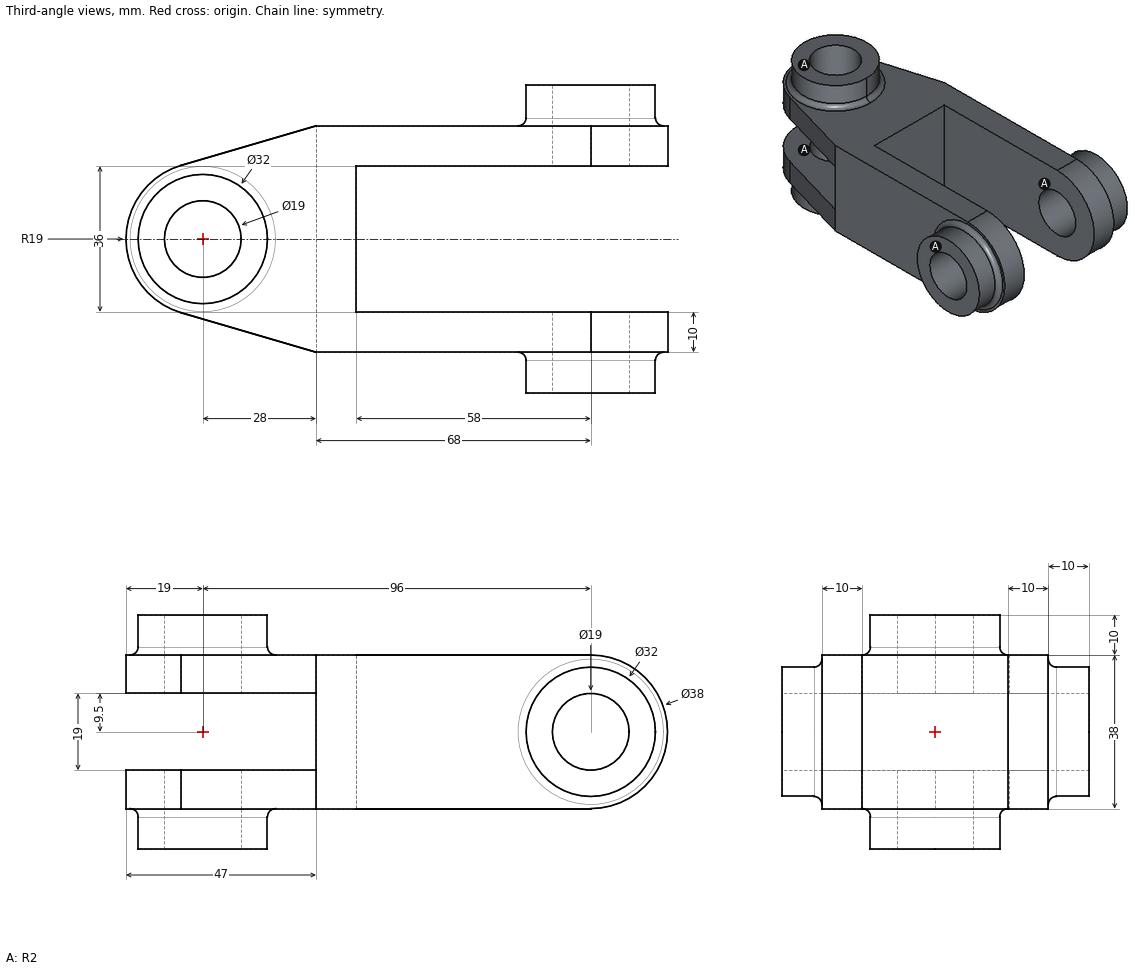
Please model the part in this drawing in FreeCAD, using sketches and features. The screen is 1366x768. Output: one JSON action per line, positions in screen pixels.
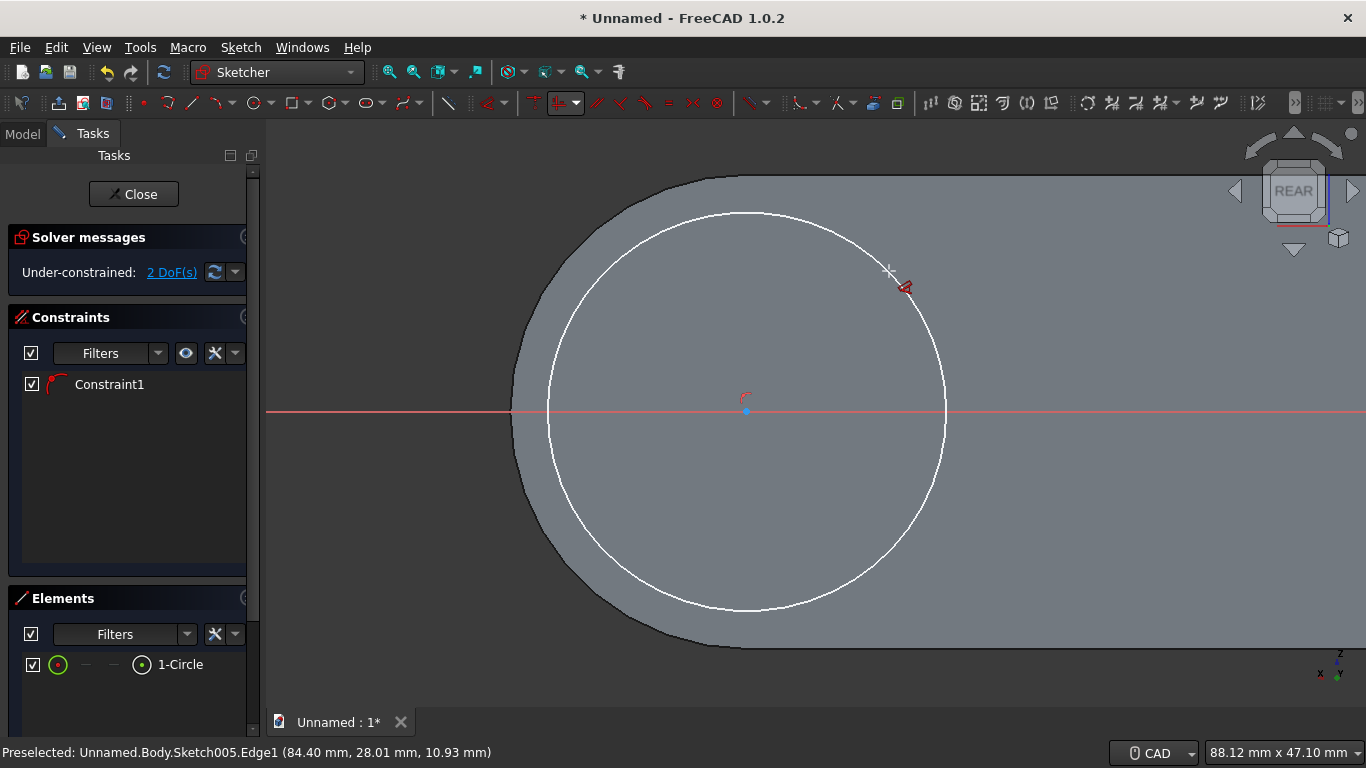
{"action": "left_click", "coordinate": [887, 270]}
{"action": "left_click", "coordinate": [909, 247]}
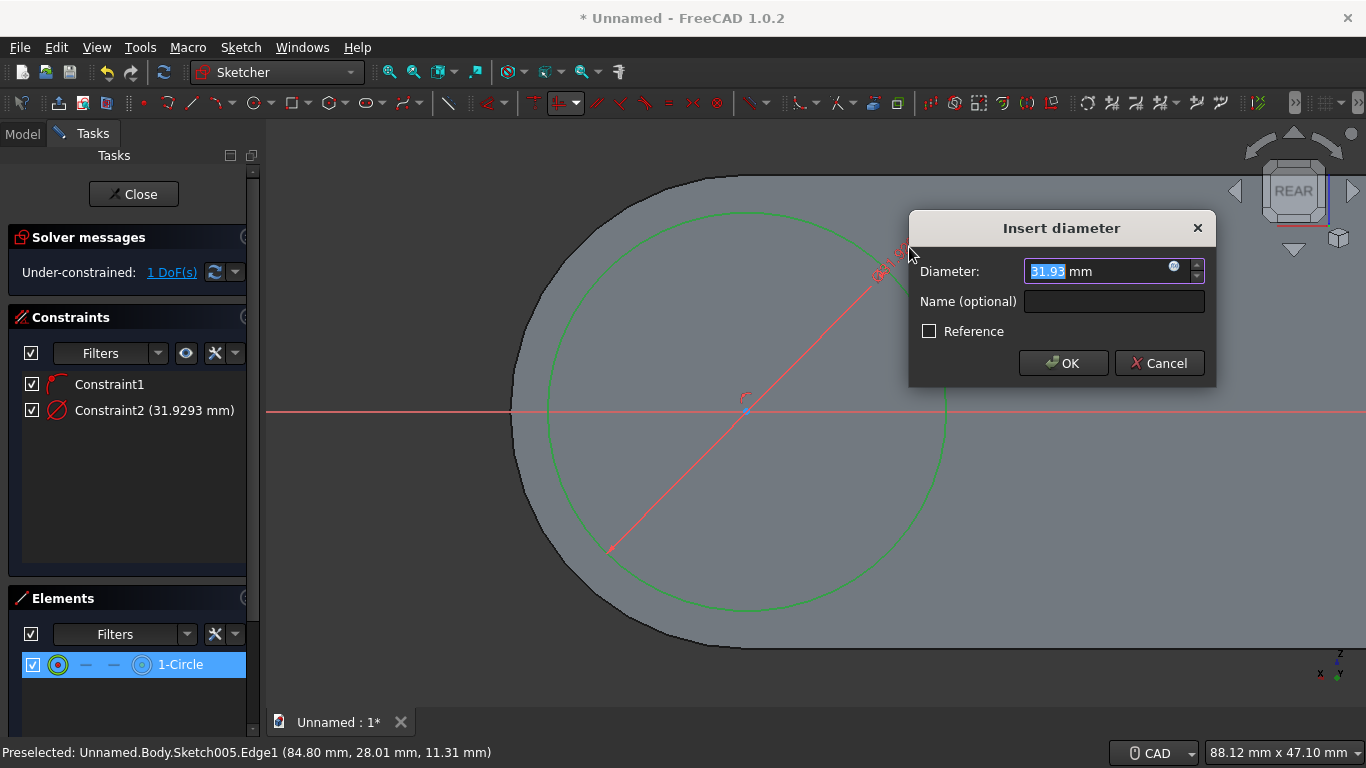
{"action": "type", "text": "32"}
{"action": "key", "text": "Return"}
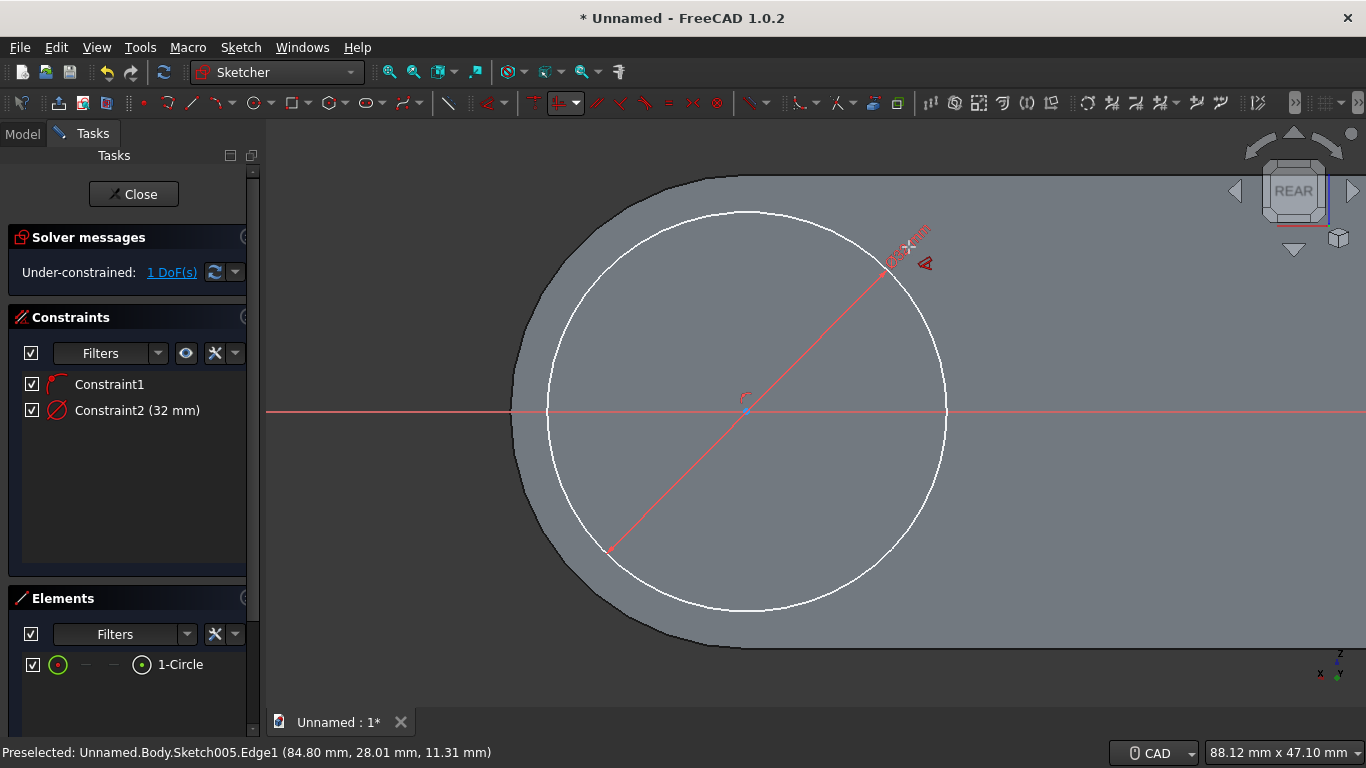
{"action": "left_click", "coordinate": [747, 412]}
{"action": "left_click", "coordinate": [974, 446]}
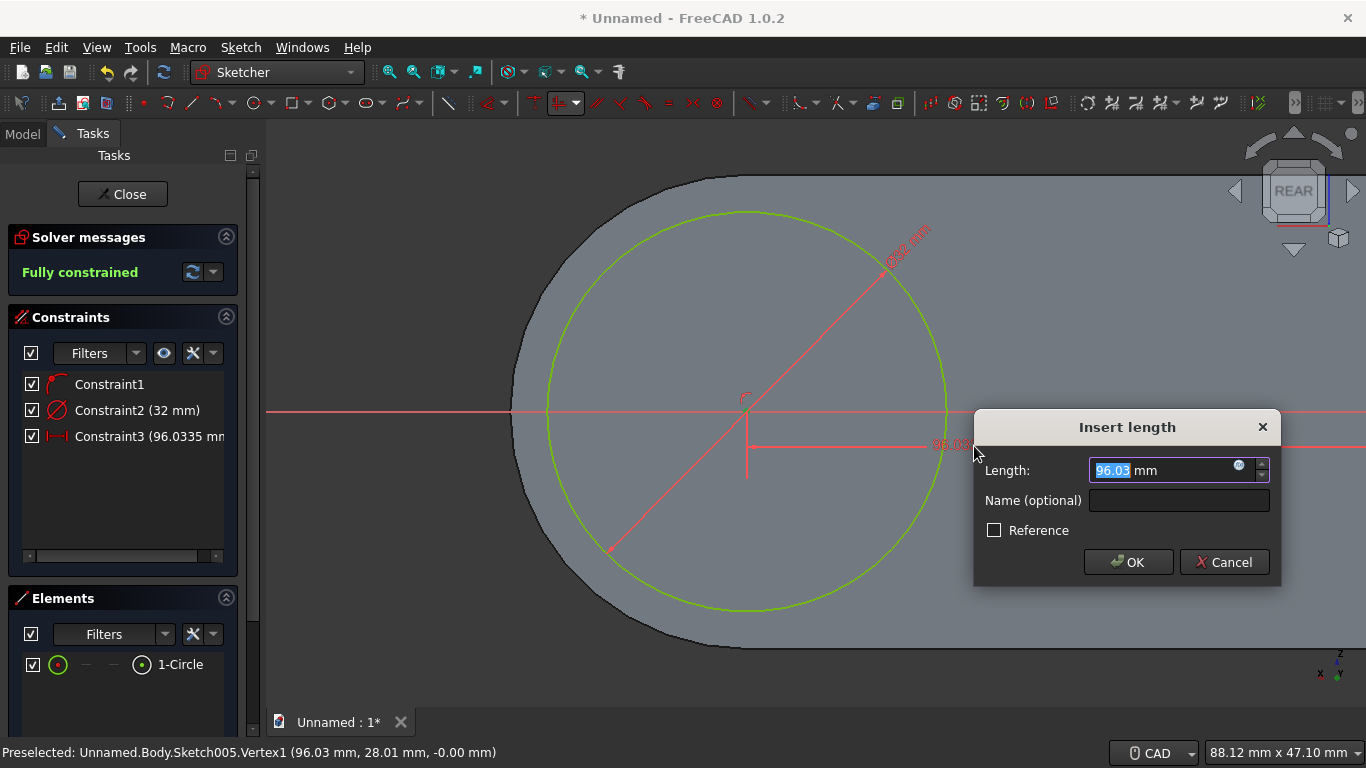
{"action": "type", "text": "96"}
{"action": "key", "text": "Return"}
{"action": "key", "text": "Escape"}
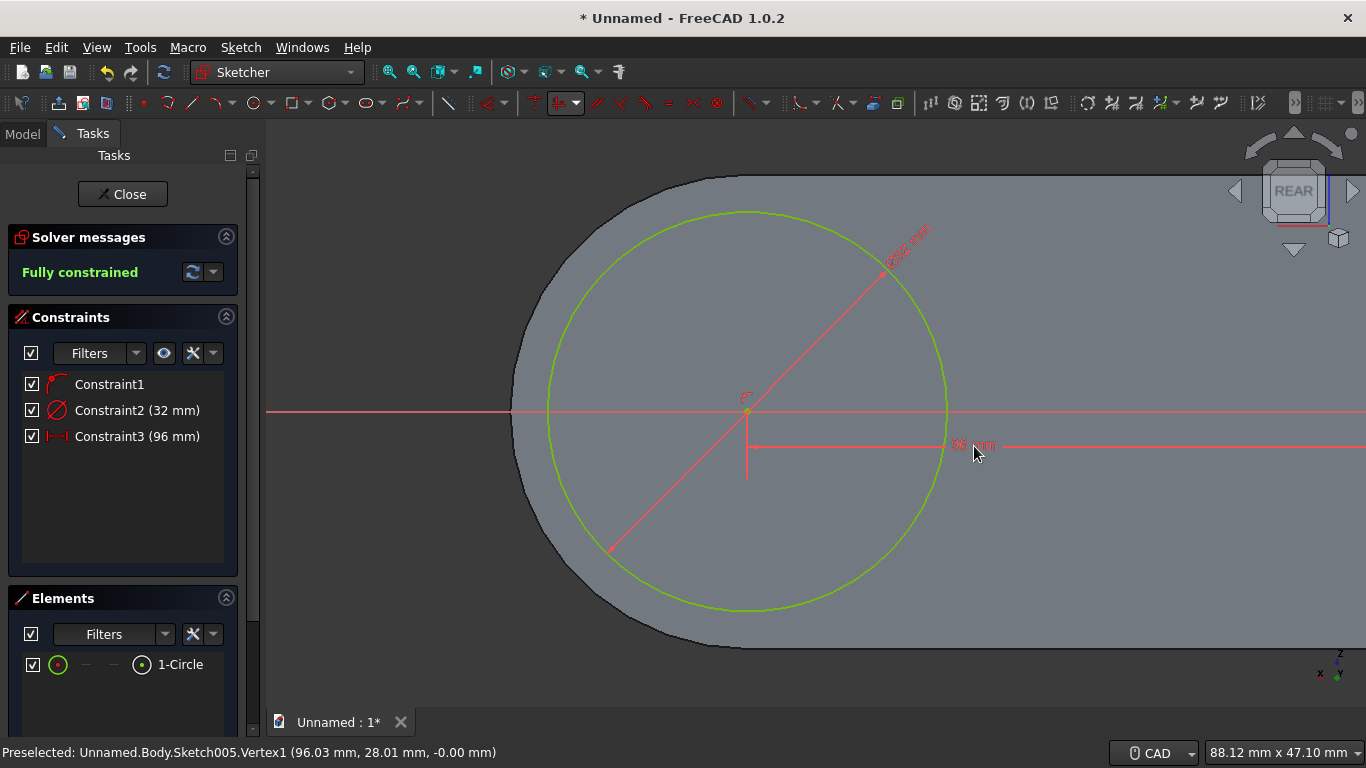
{"action": "left_click", "coordinate": [123, 194]}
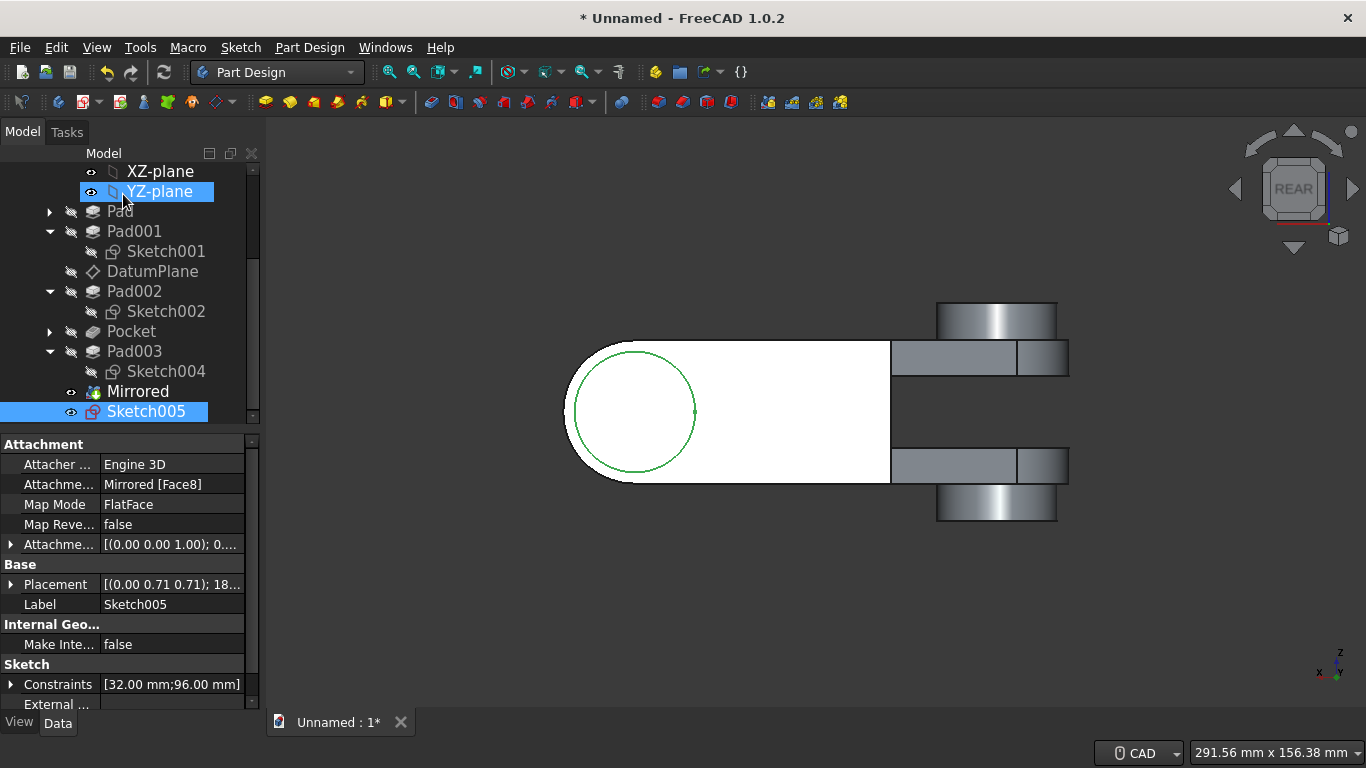
{"action": "left_click", "coordinate": [266, 102]}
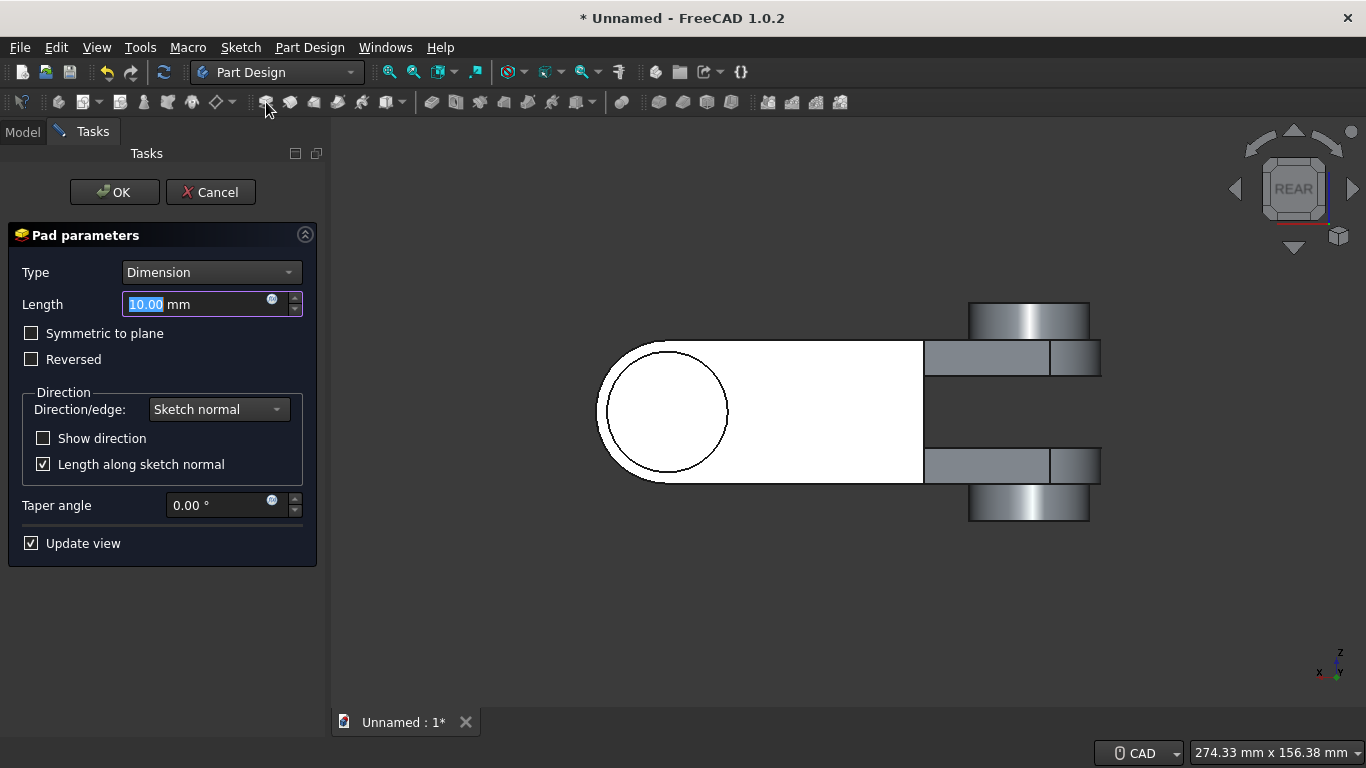
{"action": "type", "text": "10"}
{"action": "key", "text": "Tab"}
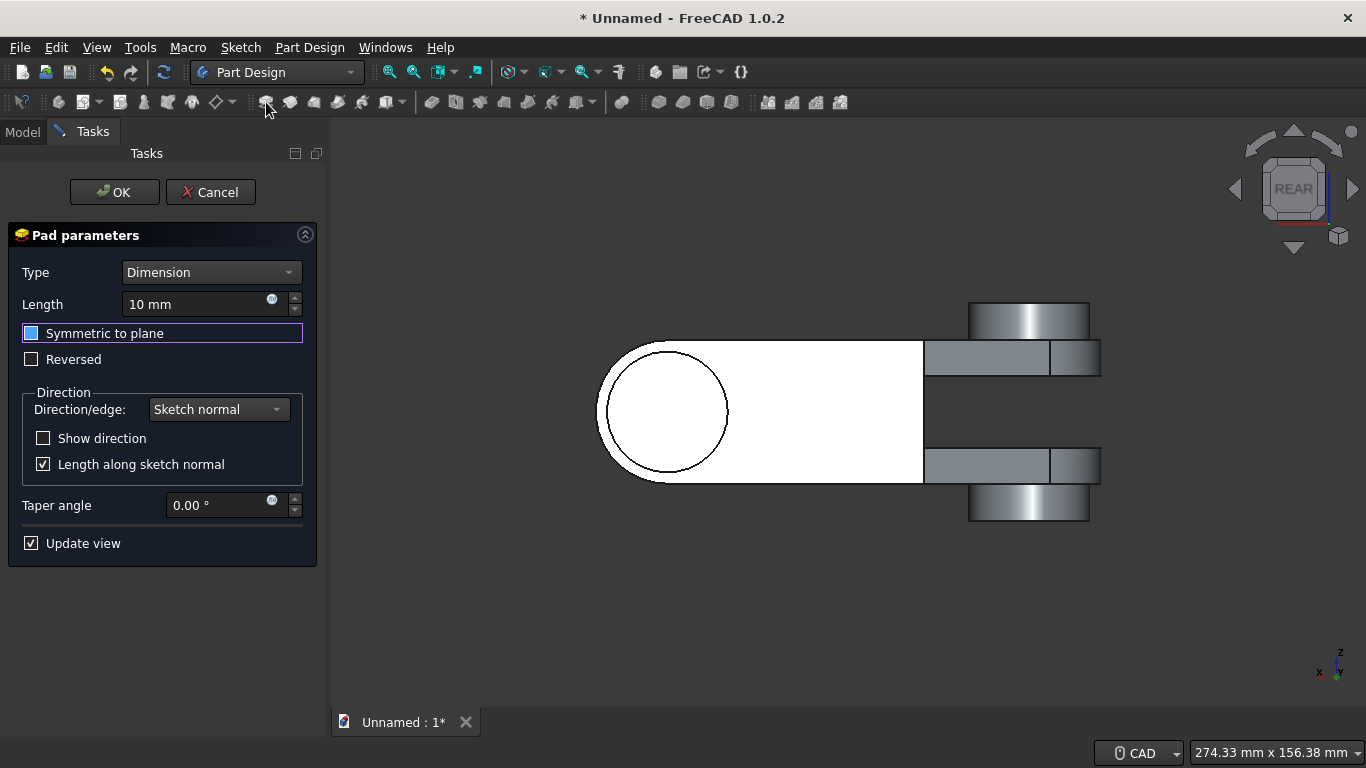
{"action": "left_click", "coordinate": [115, 192]}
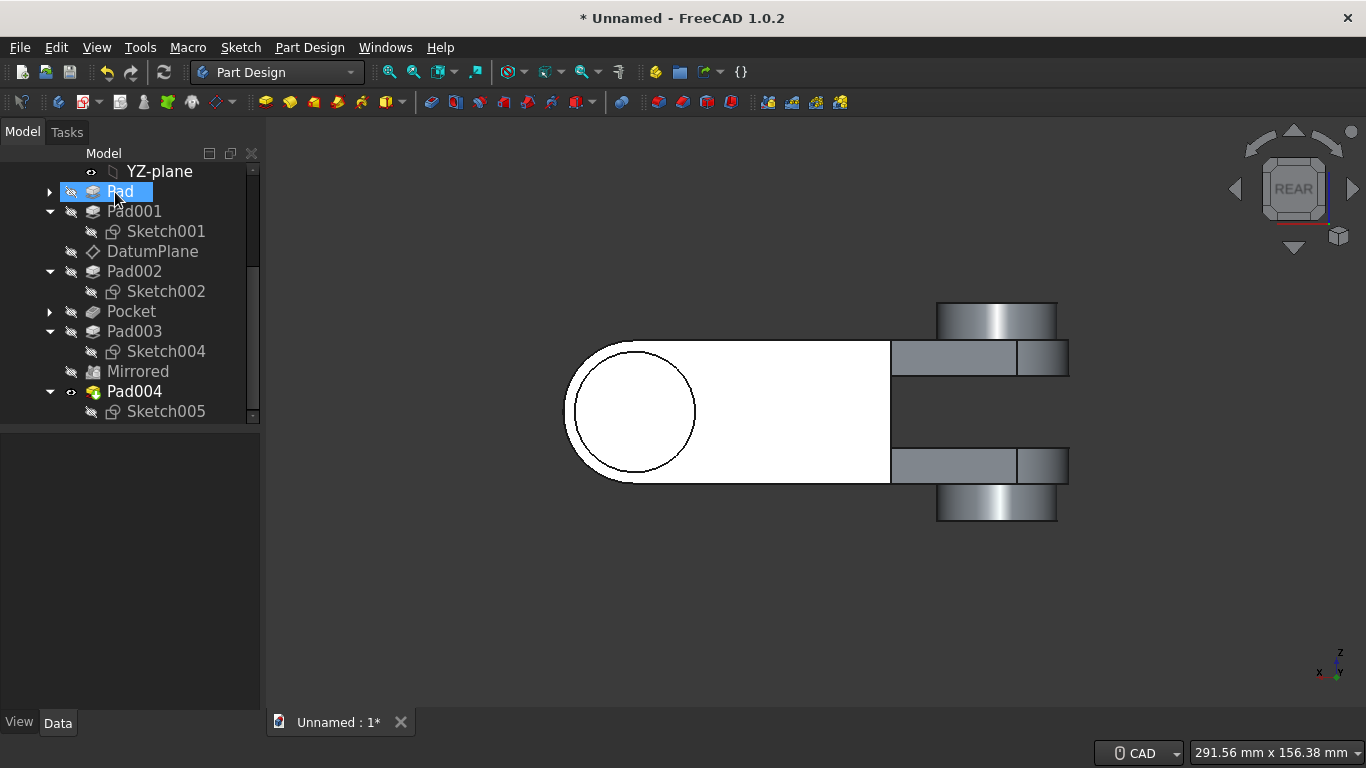
{"action": "left_click", "coordinate": [116, 392]}